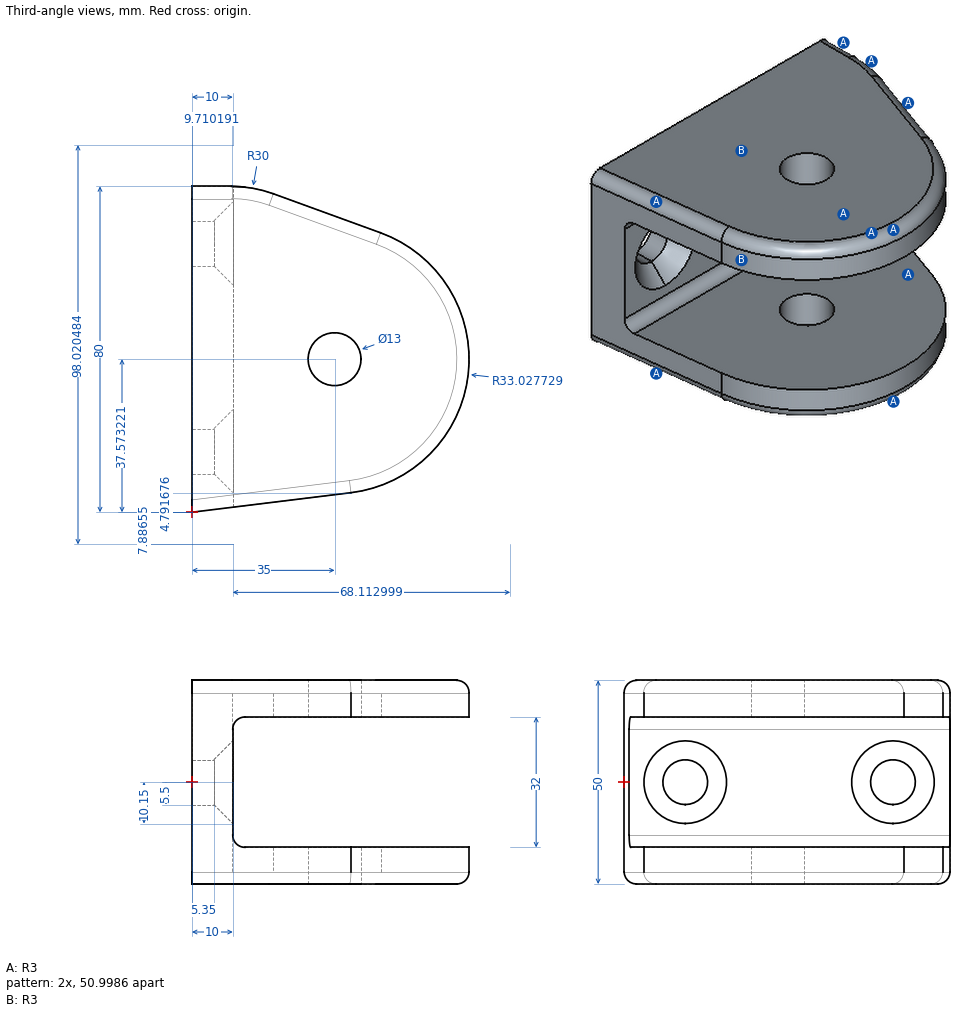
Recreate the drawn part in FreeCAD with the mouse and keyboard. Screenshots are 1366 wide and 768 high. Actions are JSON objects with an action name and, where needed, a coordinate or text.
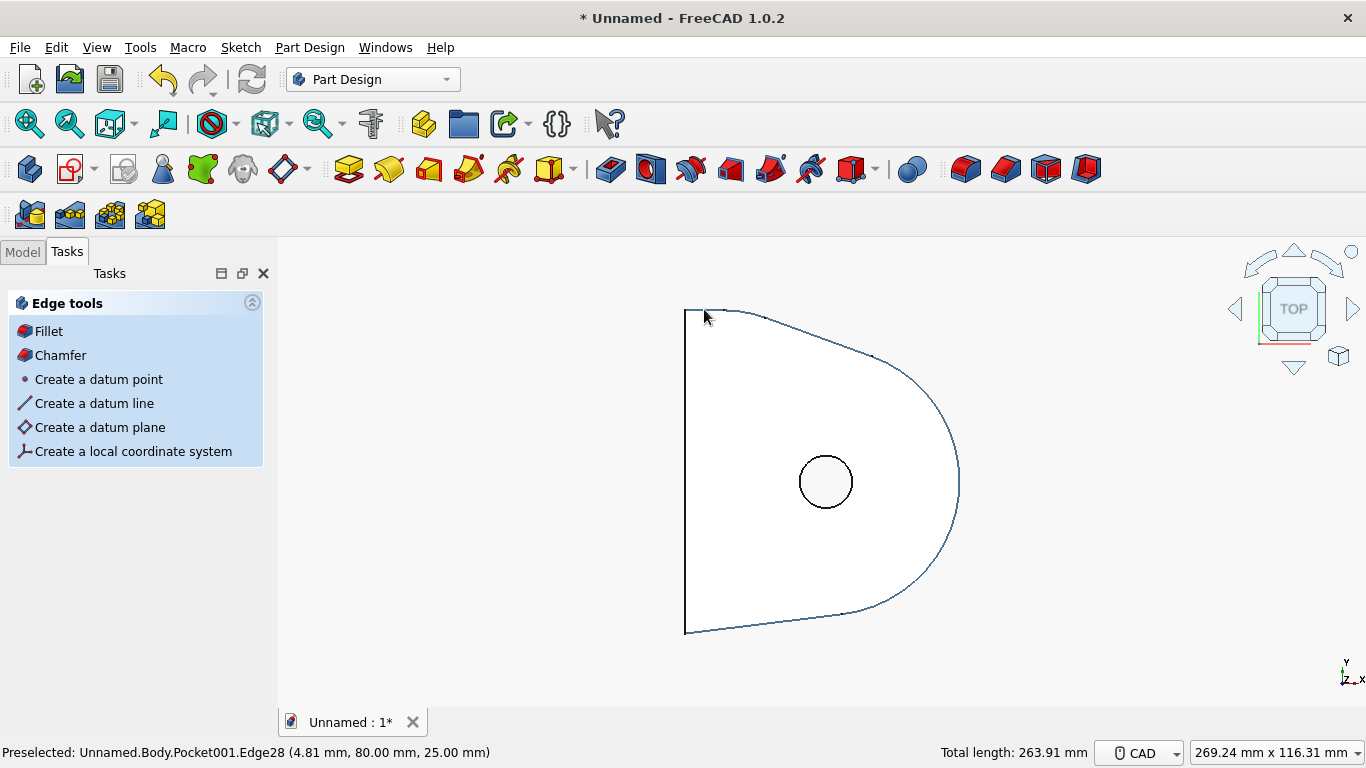
{"action": "key", "text": "1"}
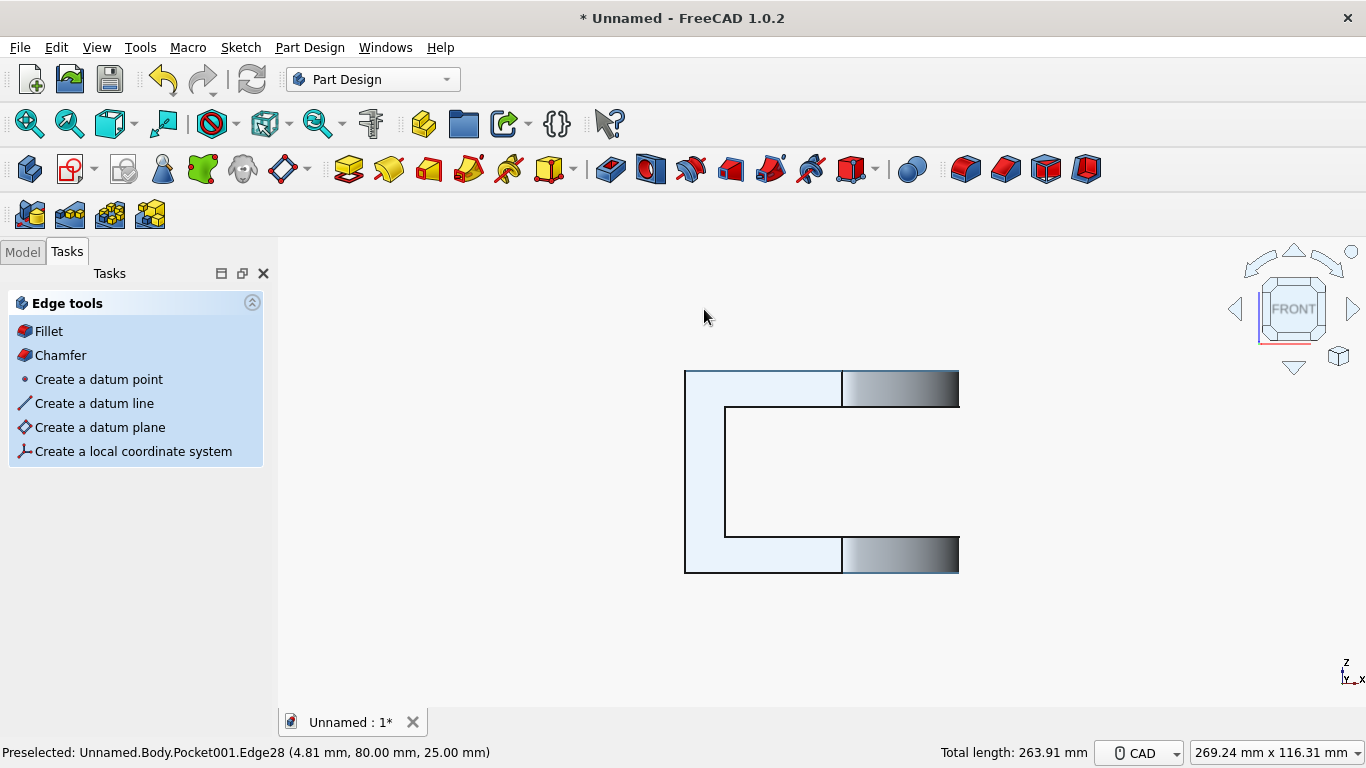
{"action": "left_click", "coordinate": [30, 124]}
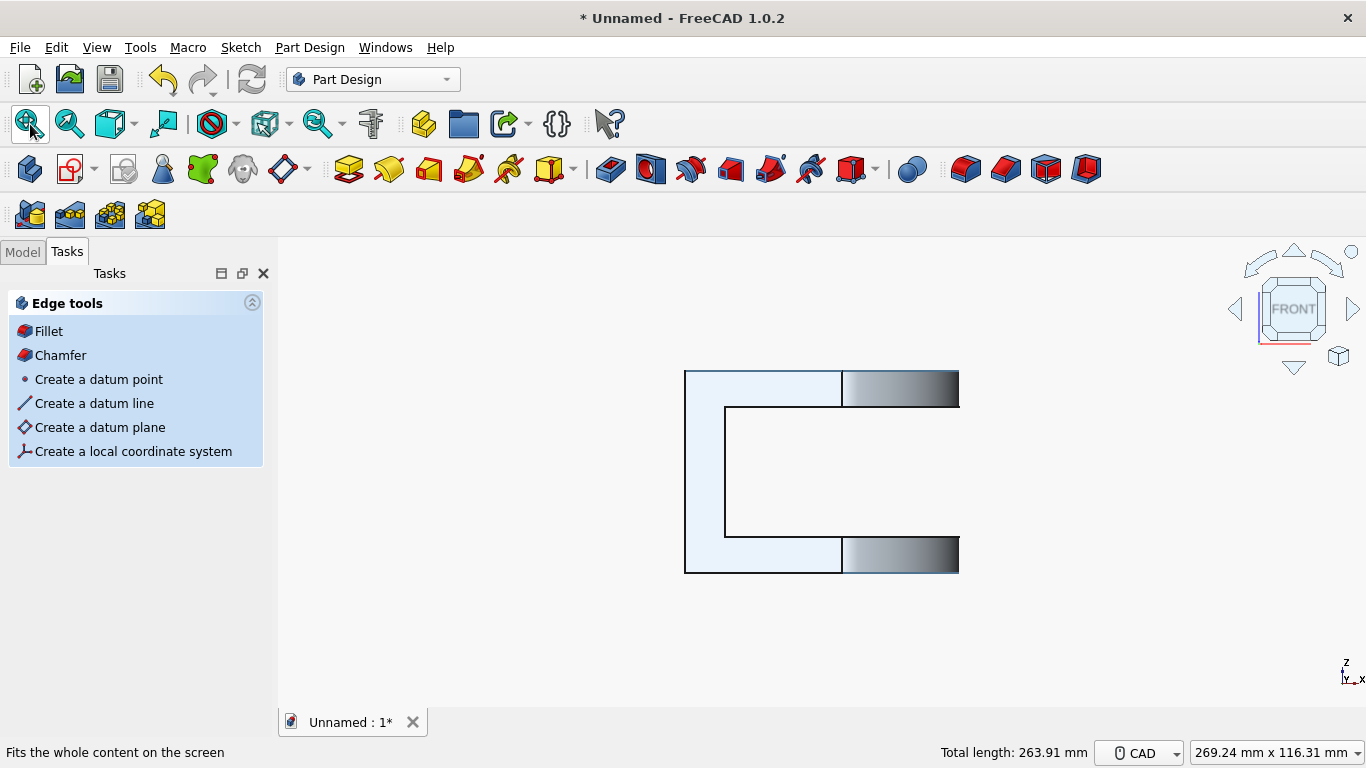
{"action": "left_click", "coordinate": [763, 572], "text": "ctrl"}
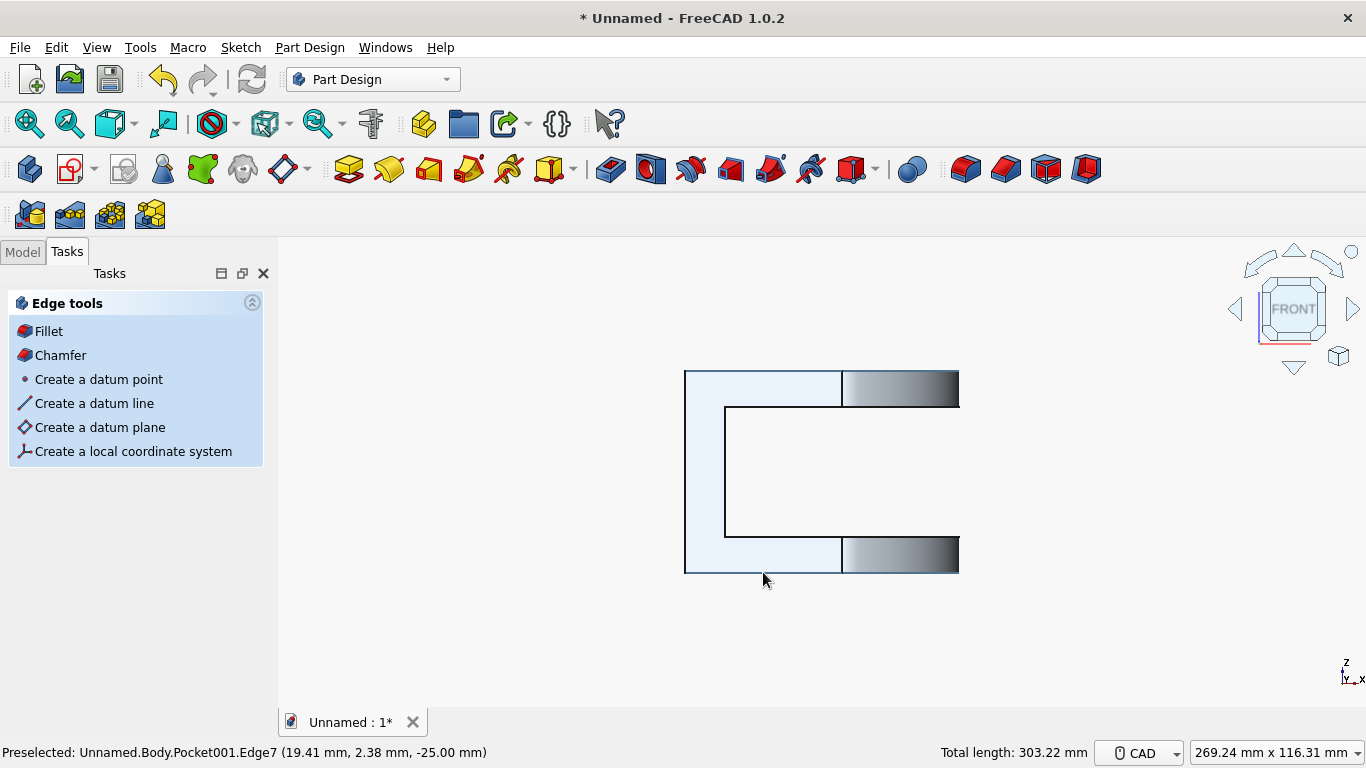
{"action": "key", "text": "3"}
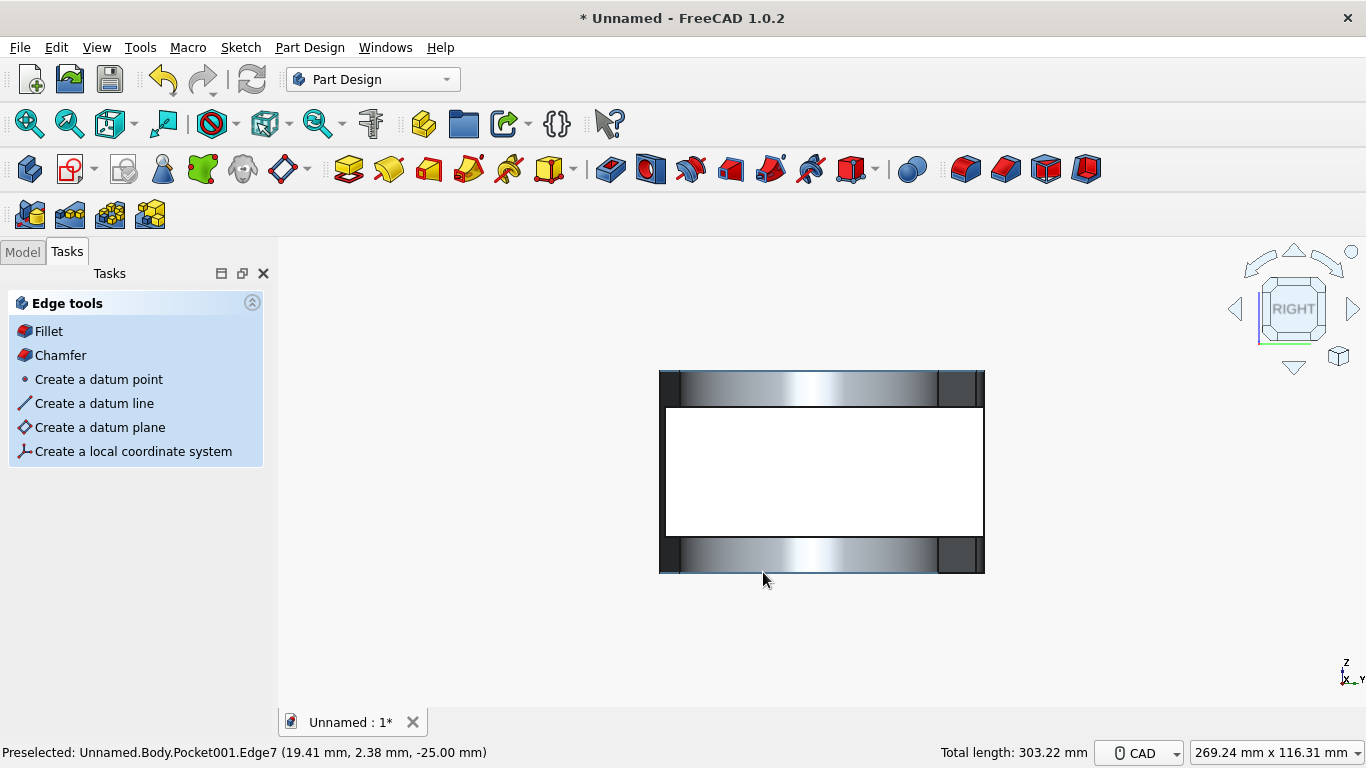
{"action": "left_click", "coordinate": [30, 124]}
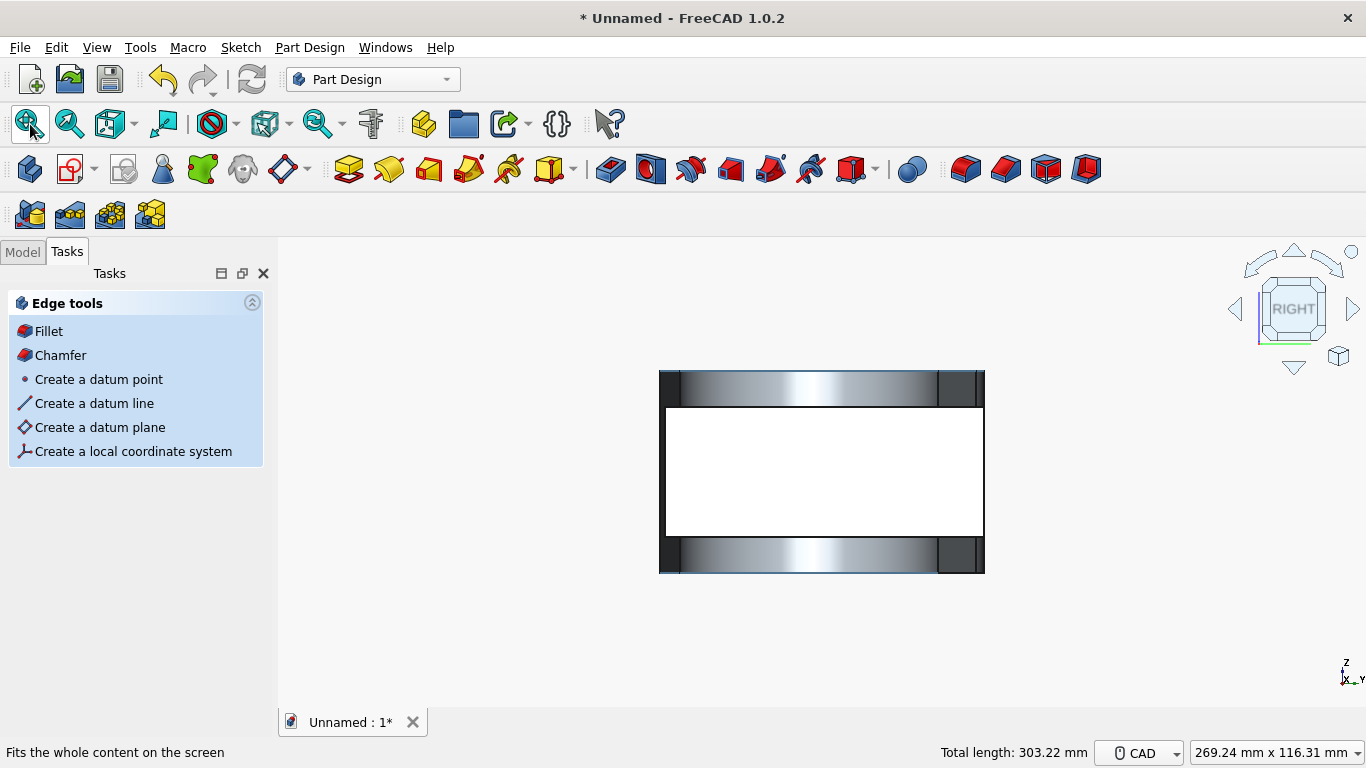
{"action": "left_click", "coordinate": [957, 572], "text": "ctrl"}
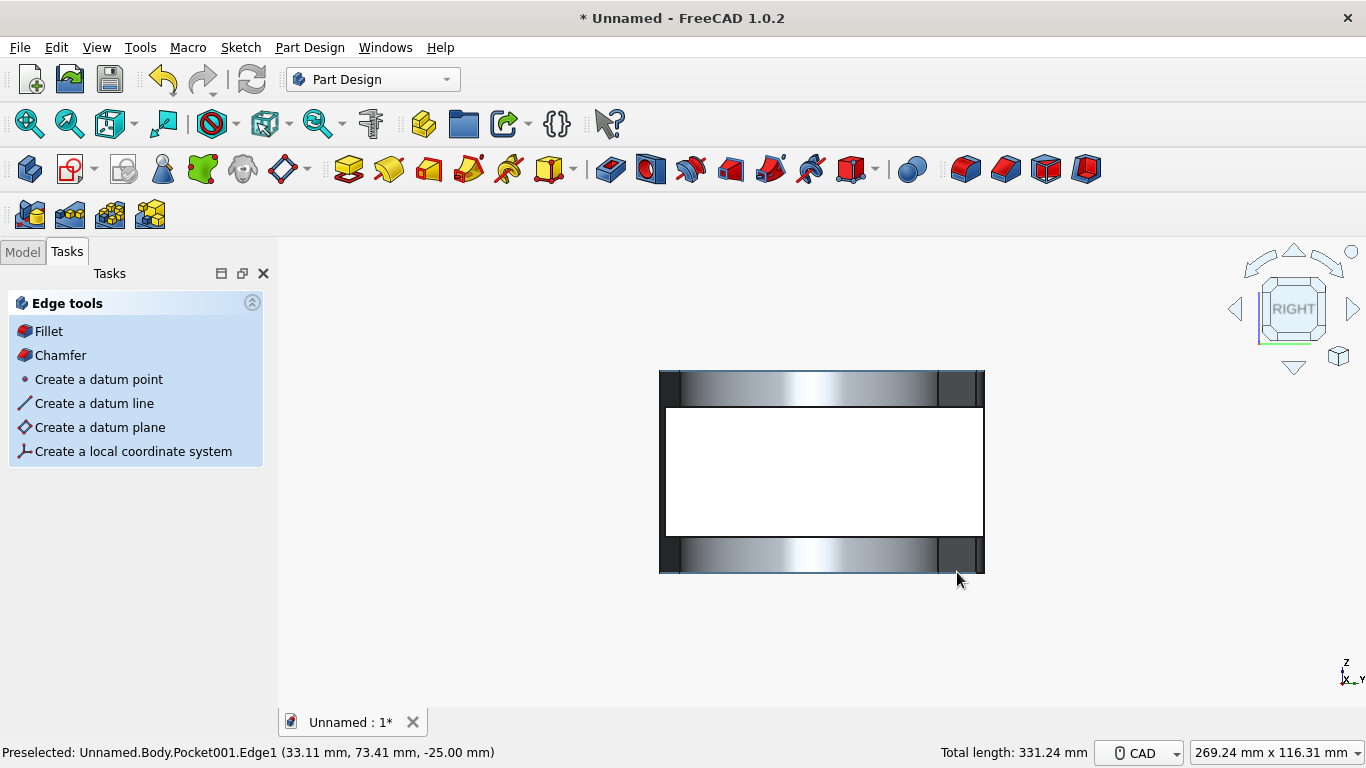
{"action": "key", "text": "5"}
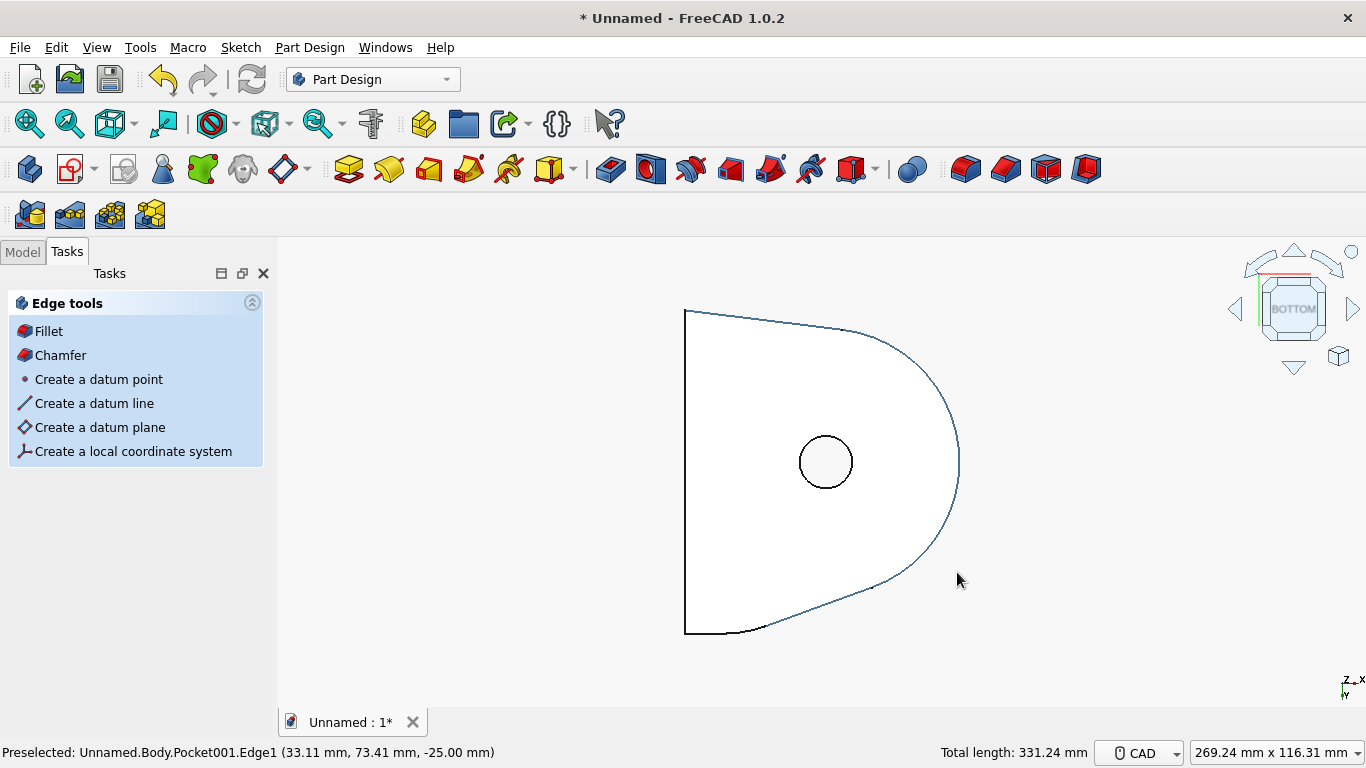
{"action": "left_click", "coordinate": [704, 633], "text": "ctrl"}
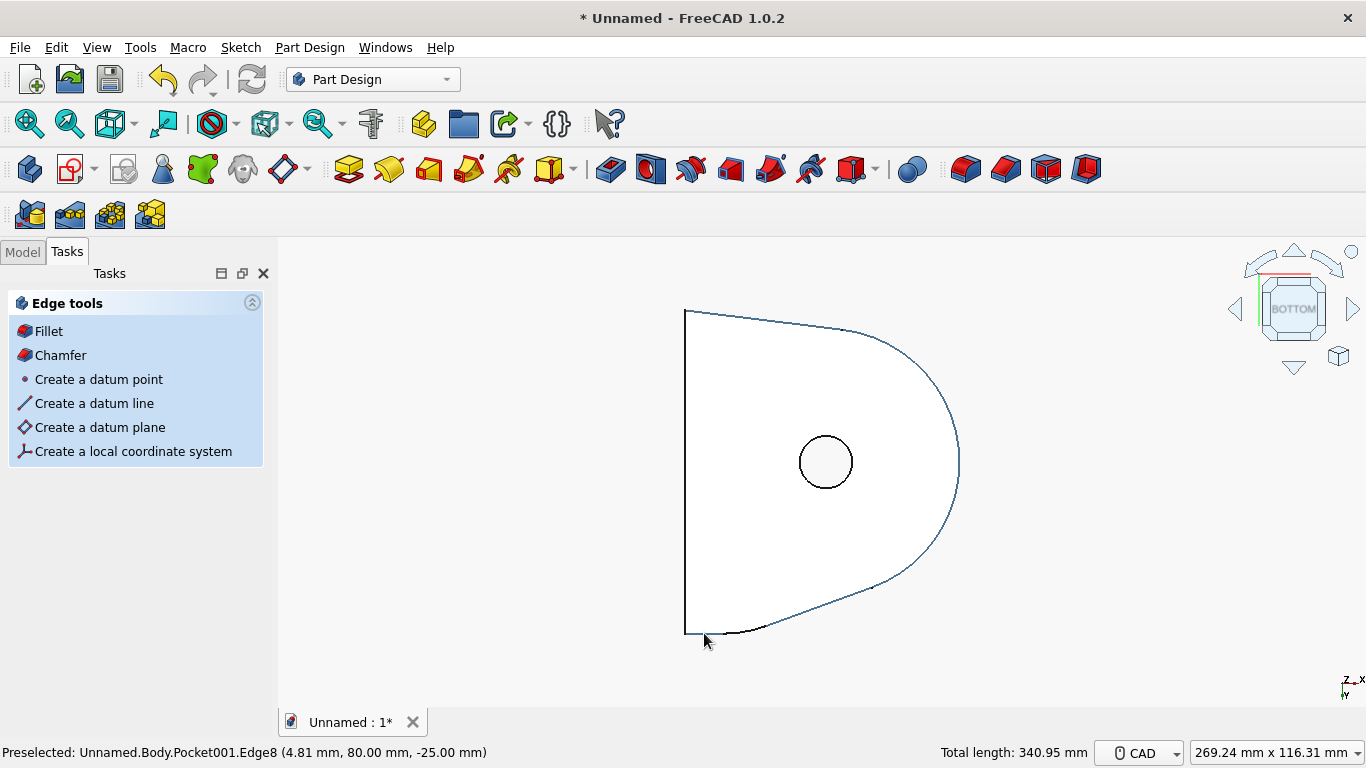
{"action": "left_click", "coordinate": [745, 631], "text": "ctrl"}